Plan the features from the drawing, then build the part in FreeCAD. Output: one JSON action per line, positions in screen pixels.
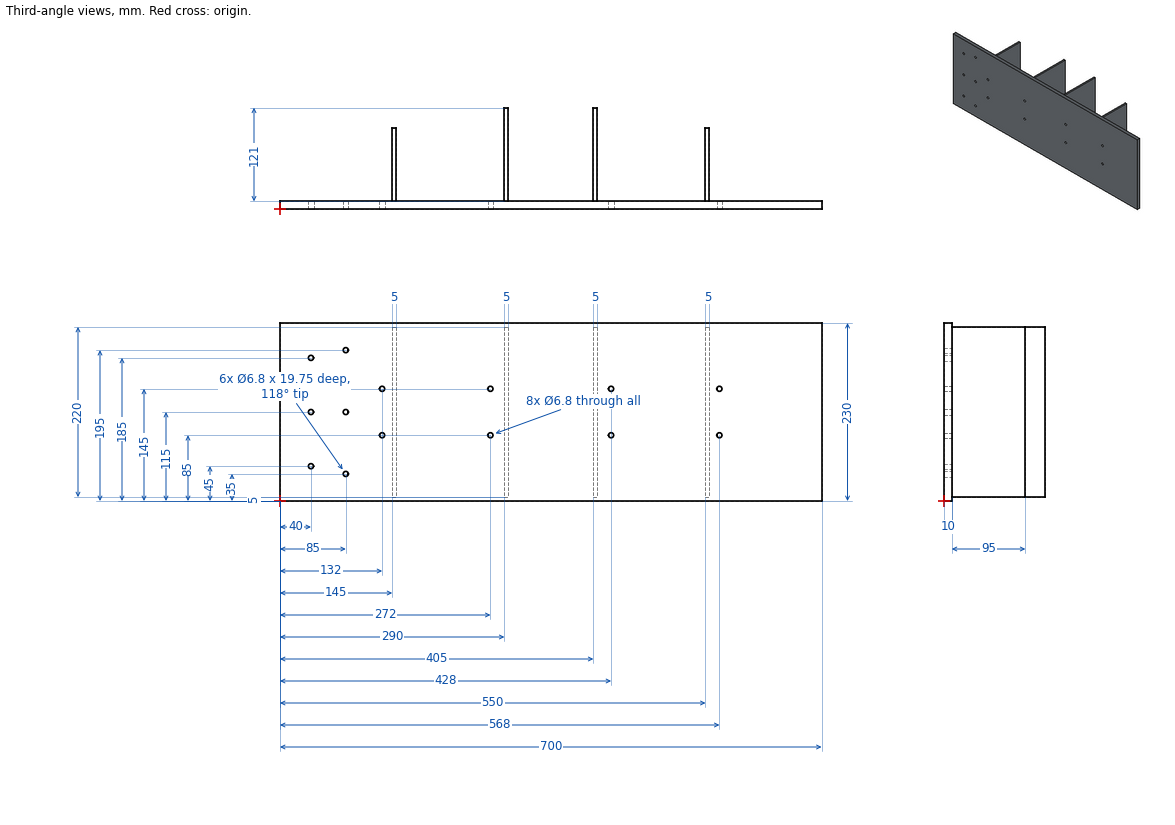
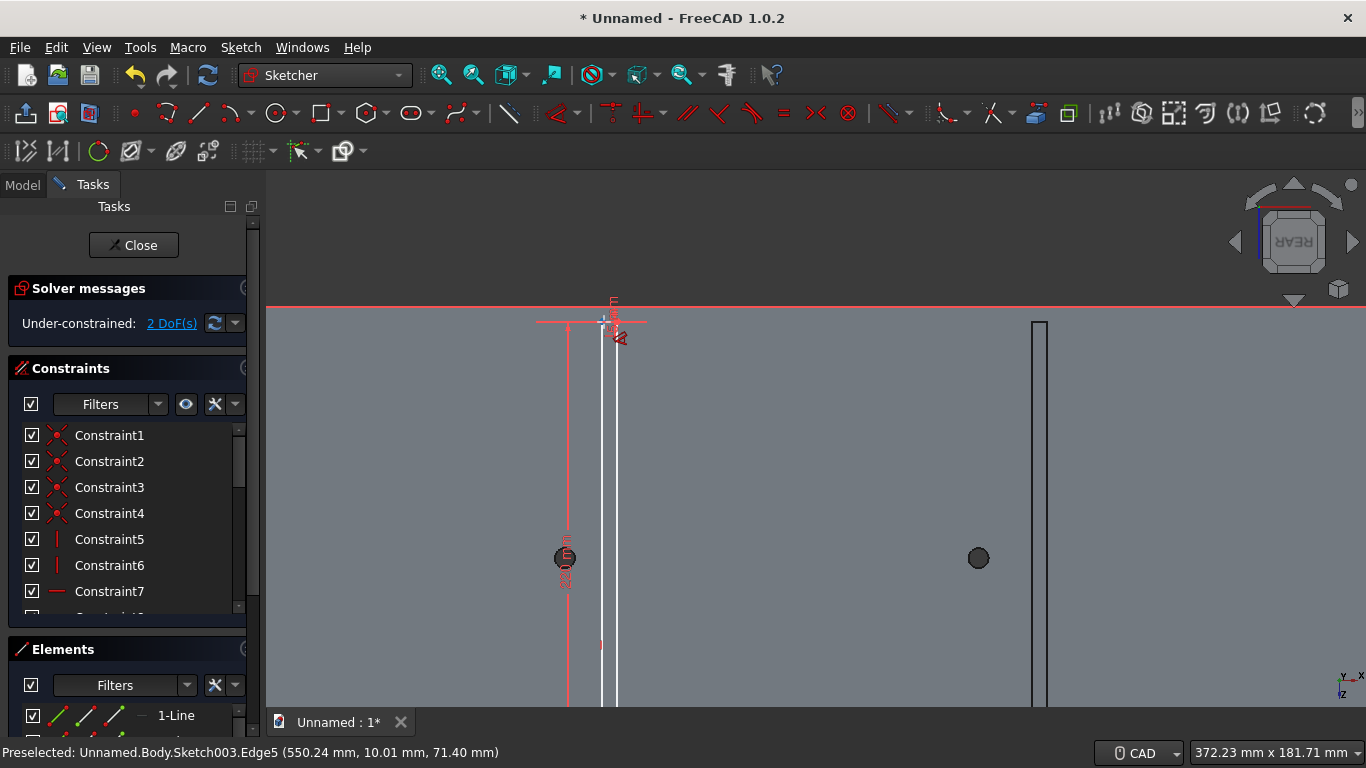
{"action": "left_click", "coordinate": [602, 322]}
{"action": "left_click", "coordinate": [448, 273]}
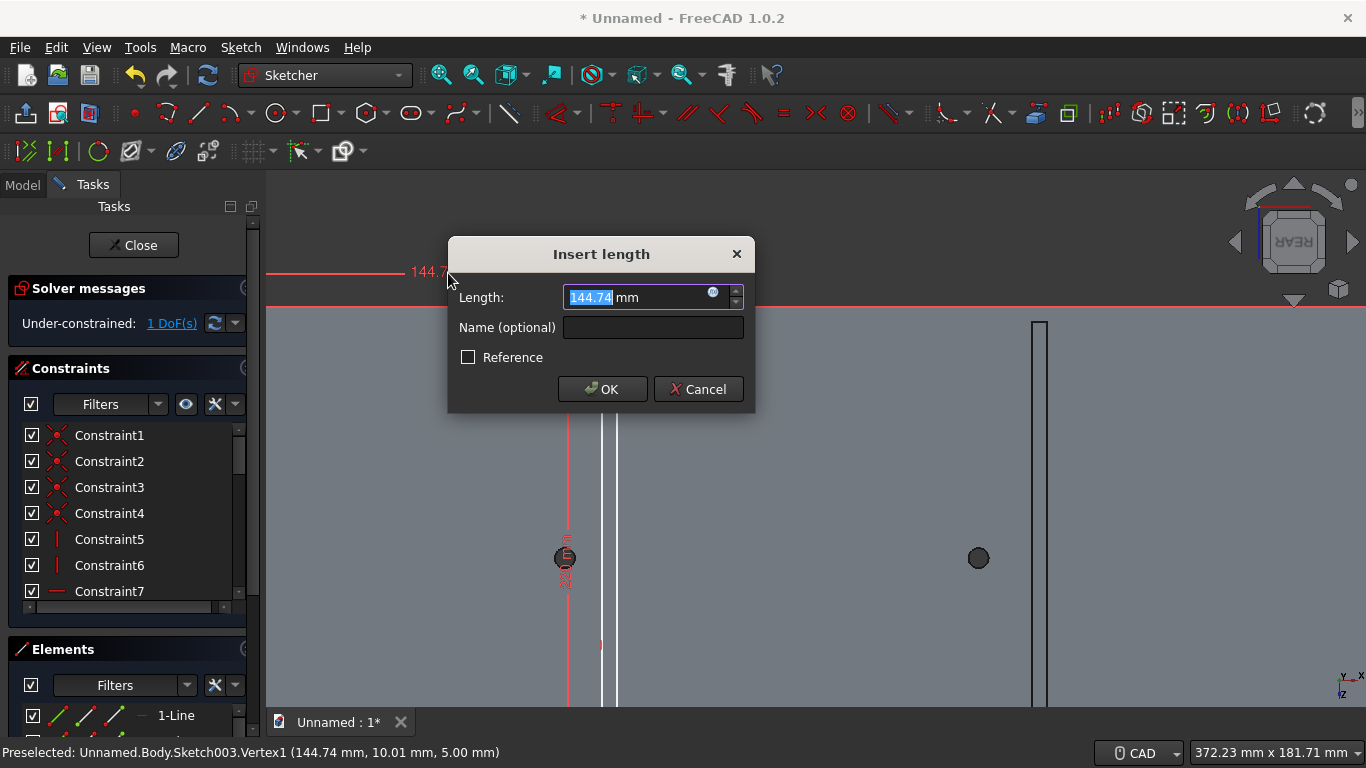
{"action": "type", "text": "145"}
{"action": "key", "text": "Return"}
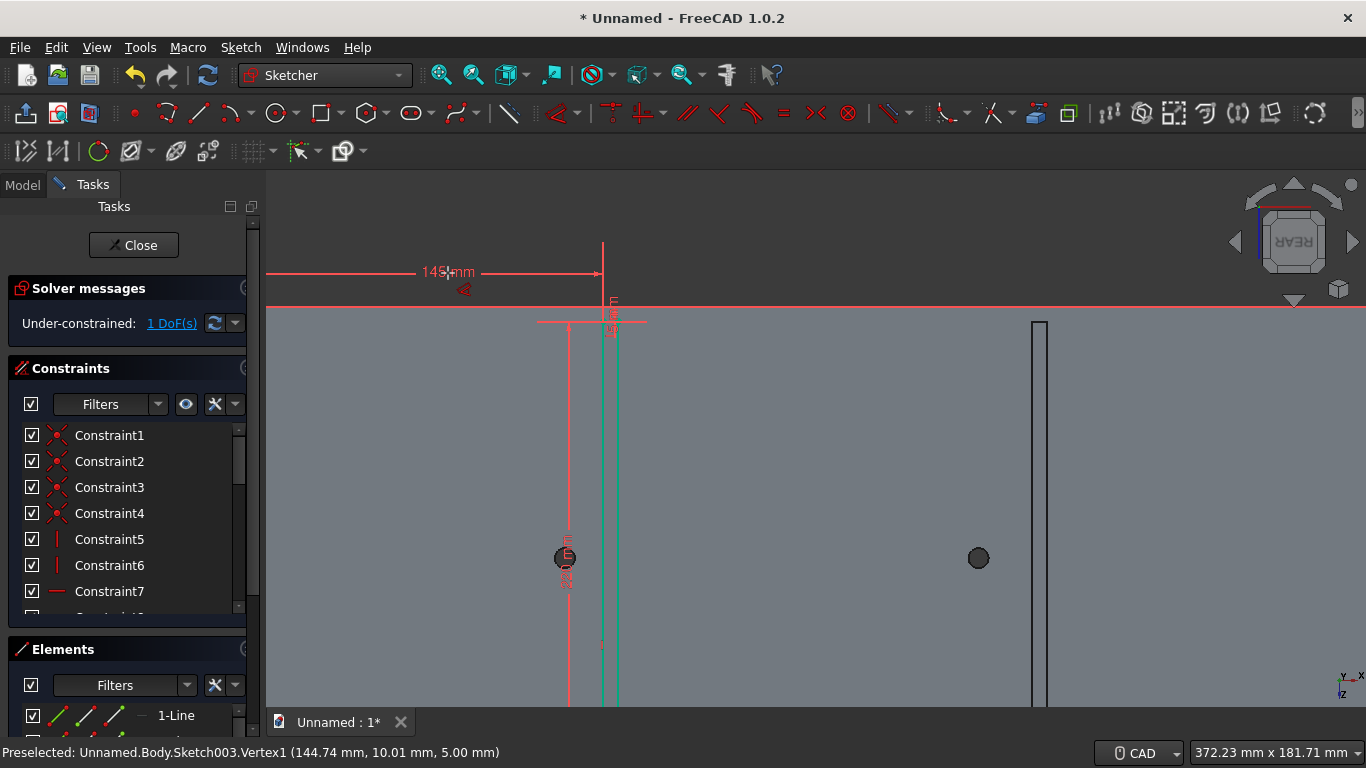
{"action": "scroll", "coordinate": [604, 322], "scroll_direction": "down", "scroll_amount": 5}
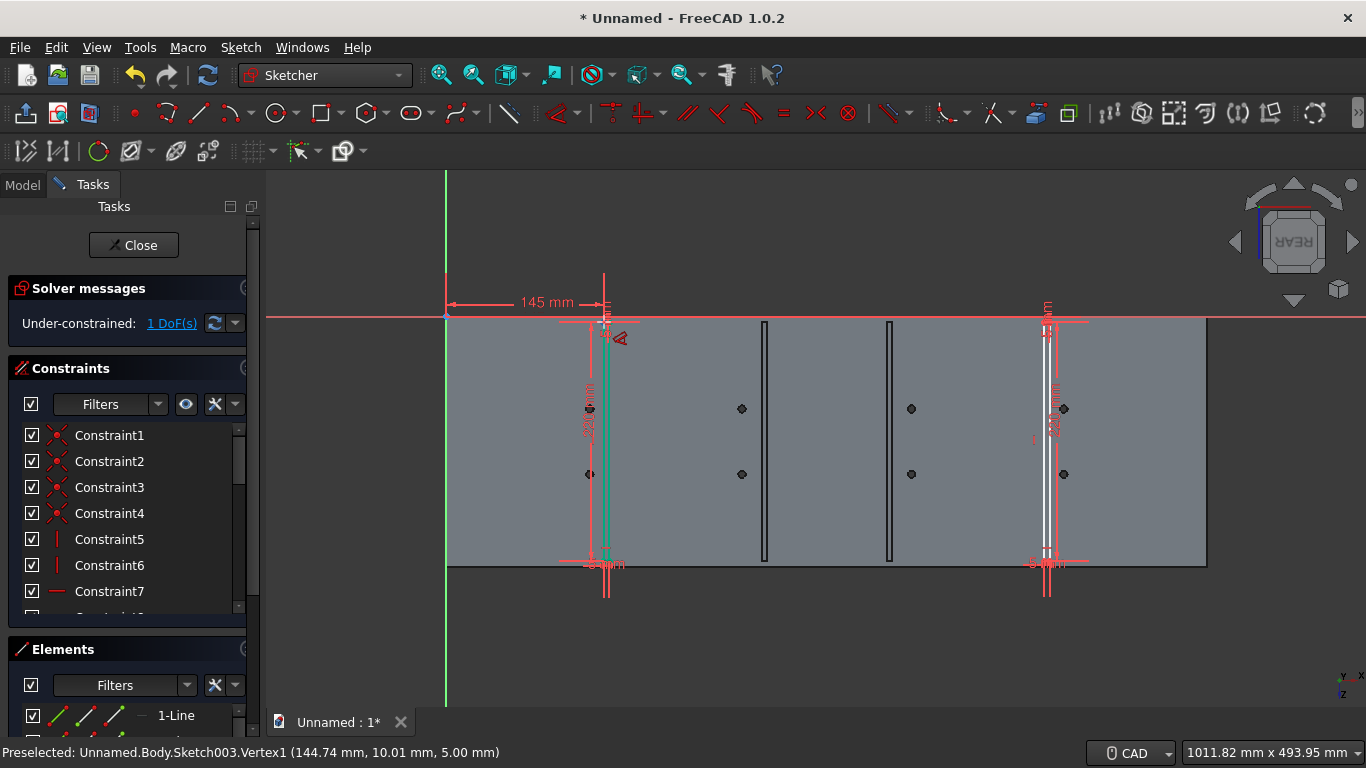
{"action": "scroll", "coordinate": [1044, 322], "scroll_direction": "up", "scroll_amount": 5}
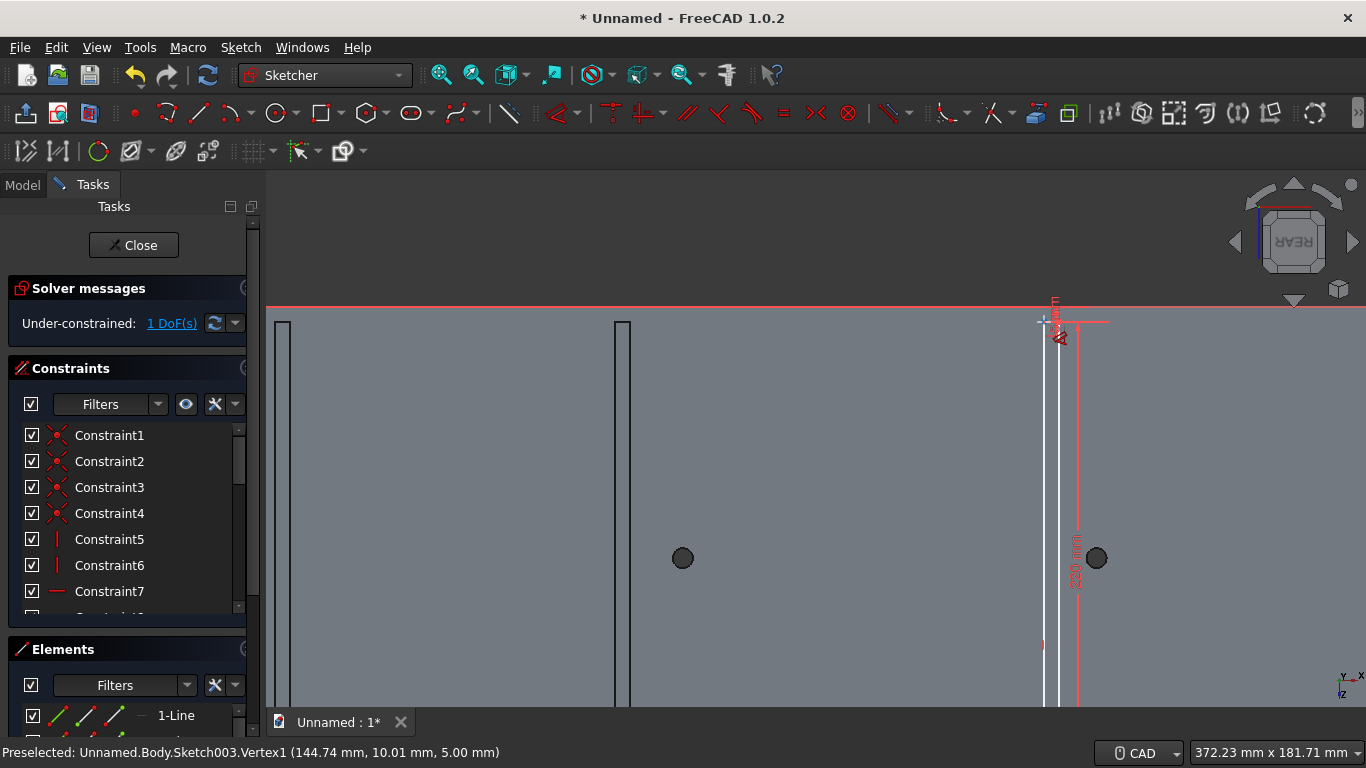
{"action": "left_click", "coordinate": [1044, 322]}
{"action": "left_click", "coordinate": [669, 273]}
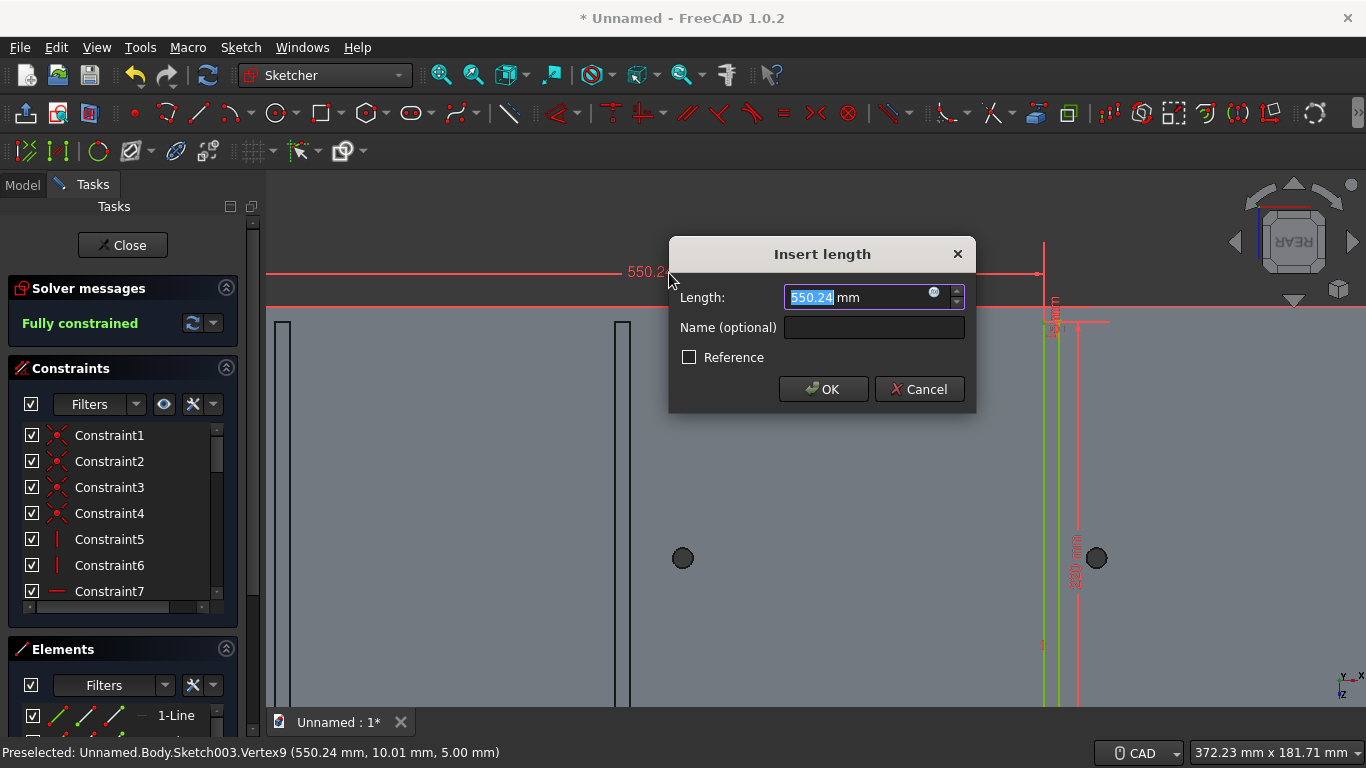
{"action": "type", "text": "550"}
{"action": "key", "text": "Return"}
{"action": "key", "text": "Escape"}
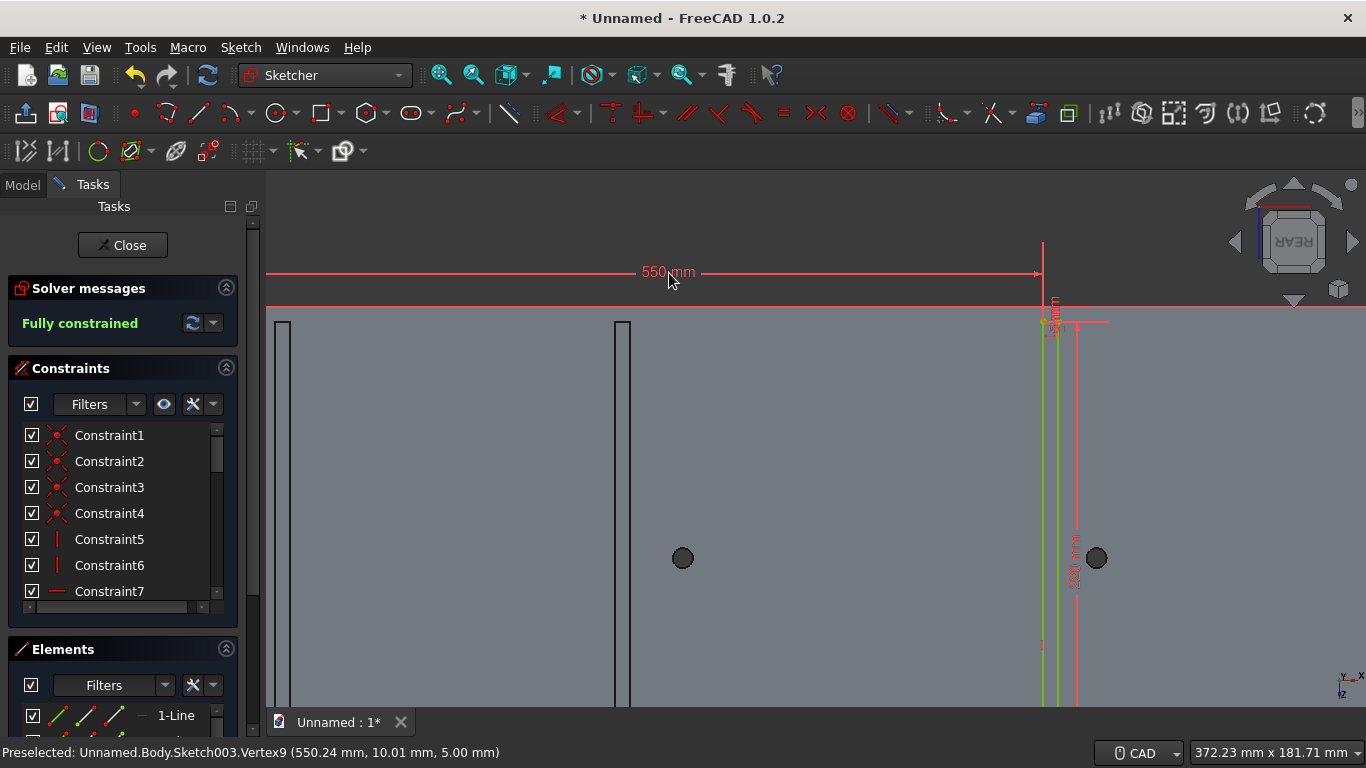
{"action": "left_click", "coordinate": [123, 245]}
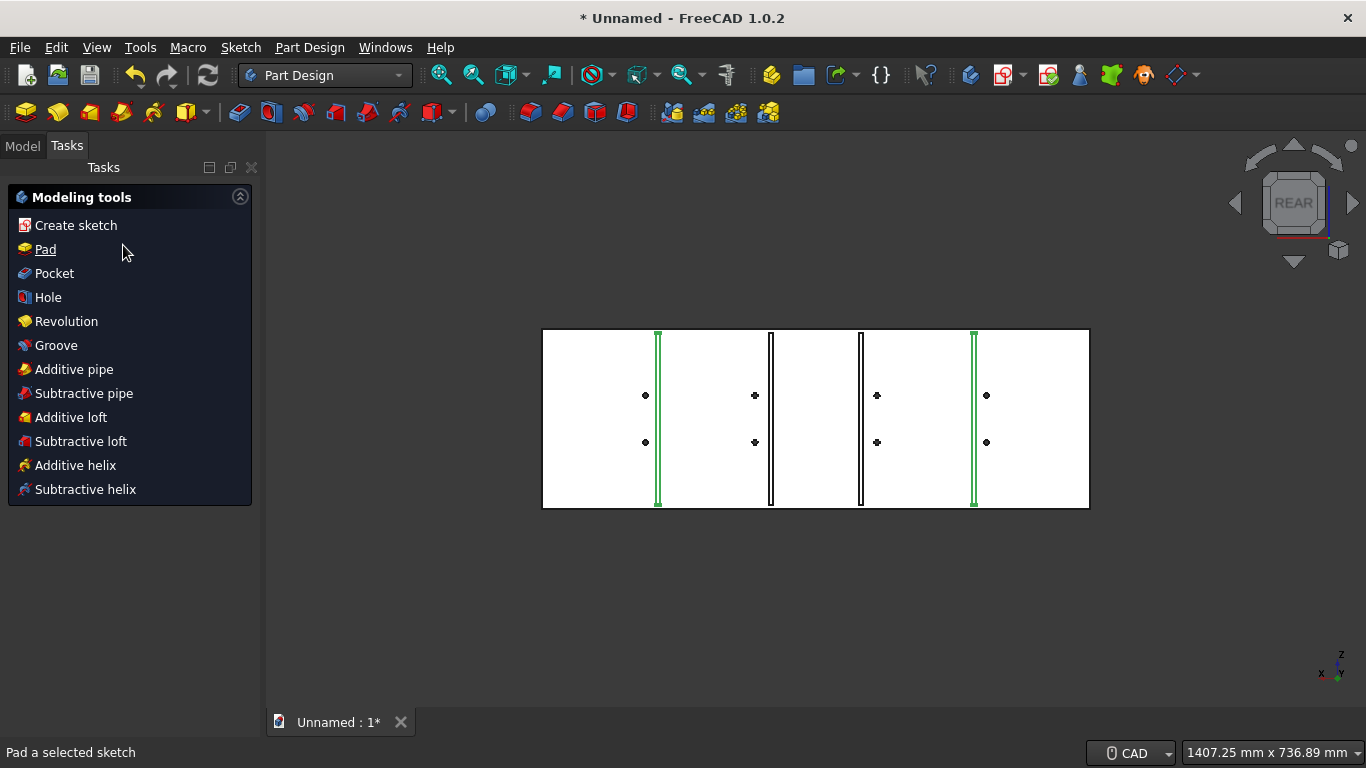
{"action": "left_click", "coordinate": [26, 112]}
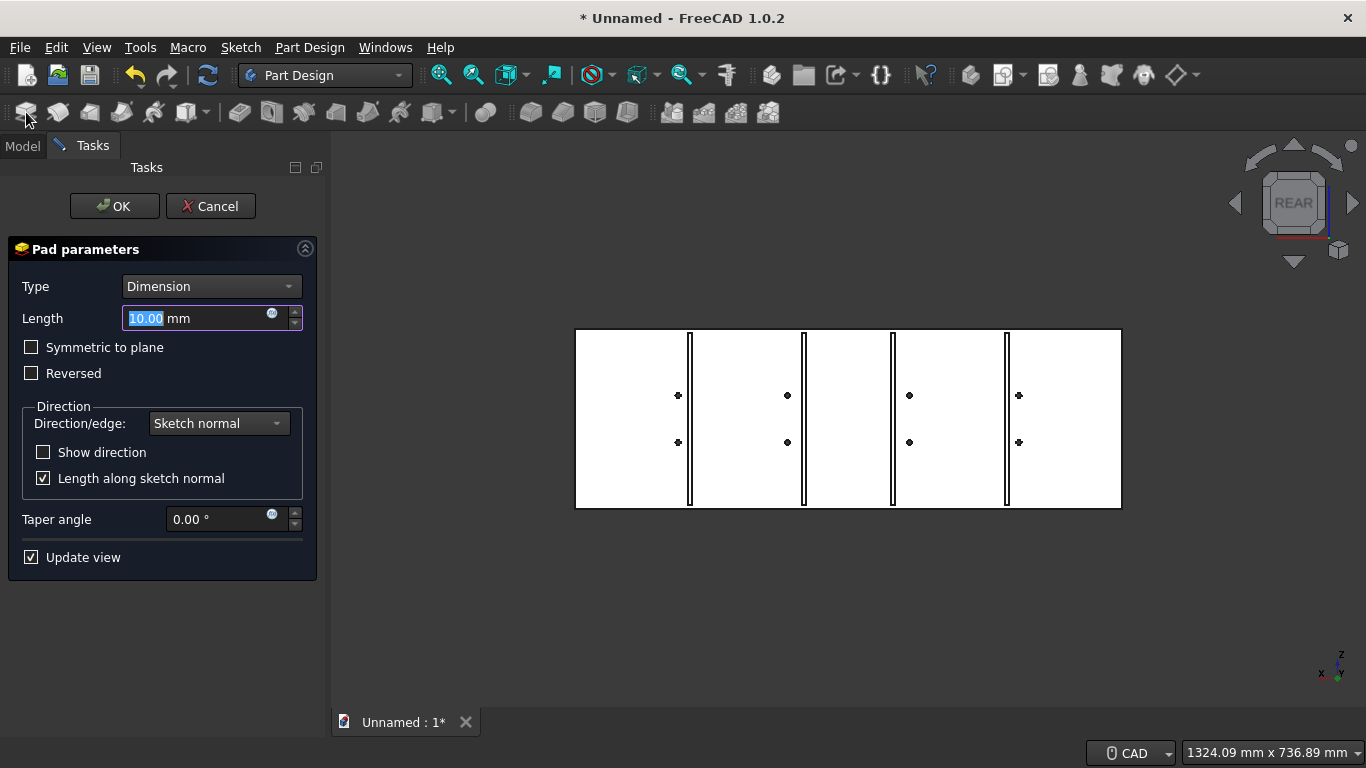
{"action": "type", "text": "95"}
{"action": "key", "text": "Tab"}